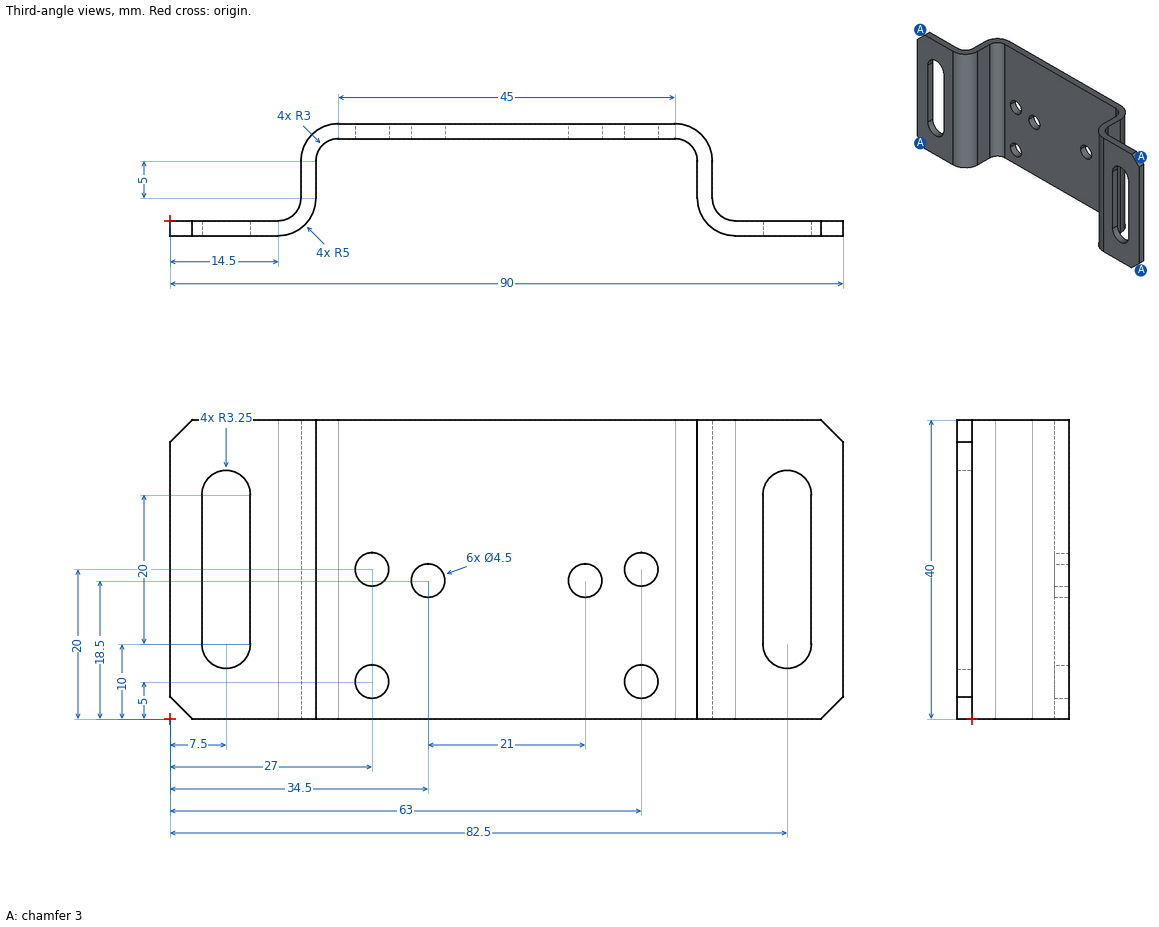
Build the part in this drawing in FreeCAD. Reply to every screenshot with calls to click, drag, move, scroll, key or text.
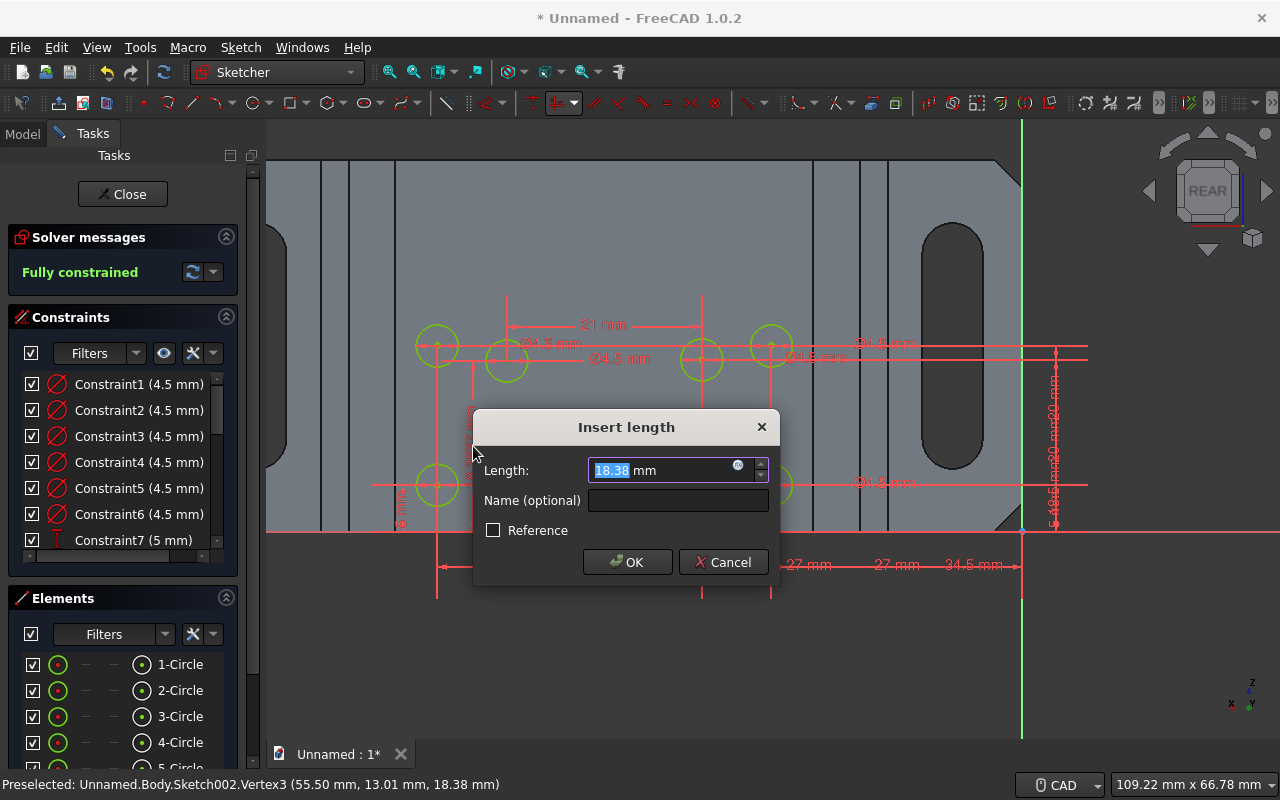
text(18.5)
key(Return)
key(Escape)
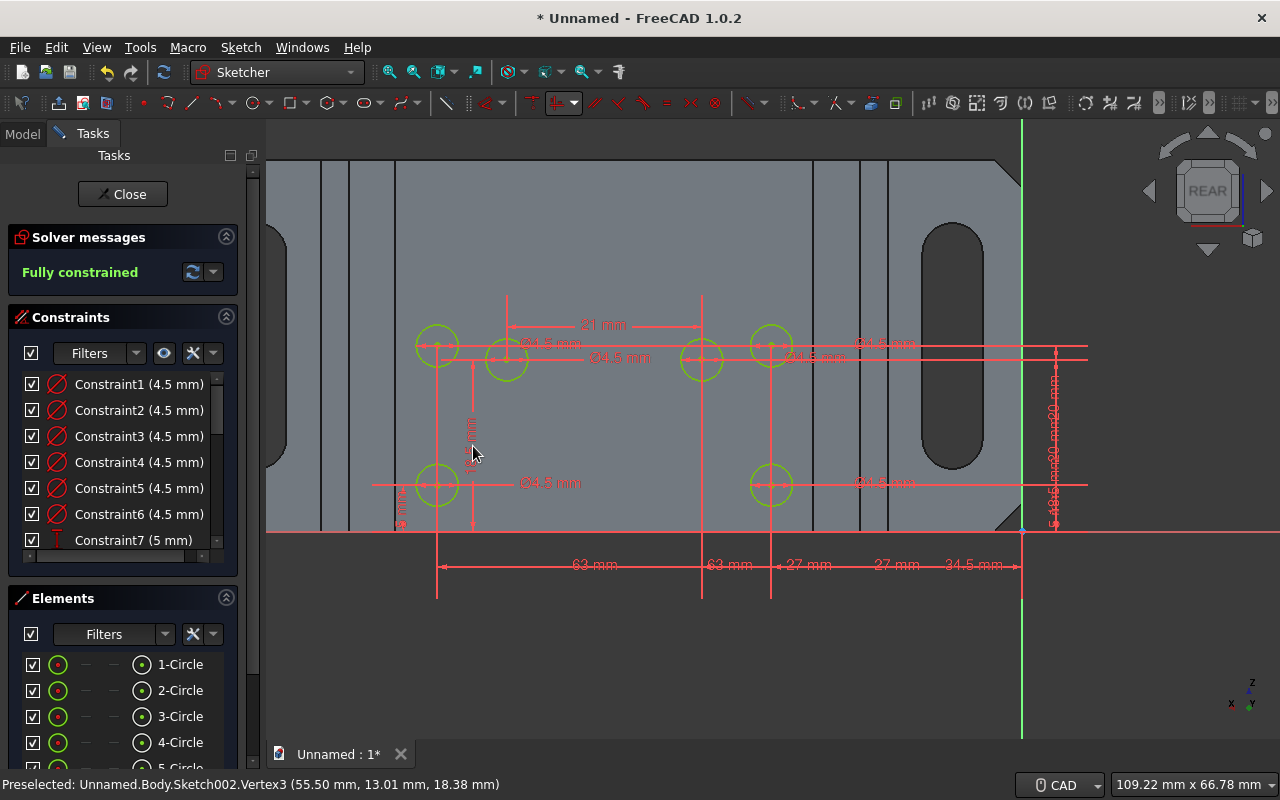
click(123, 194)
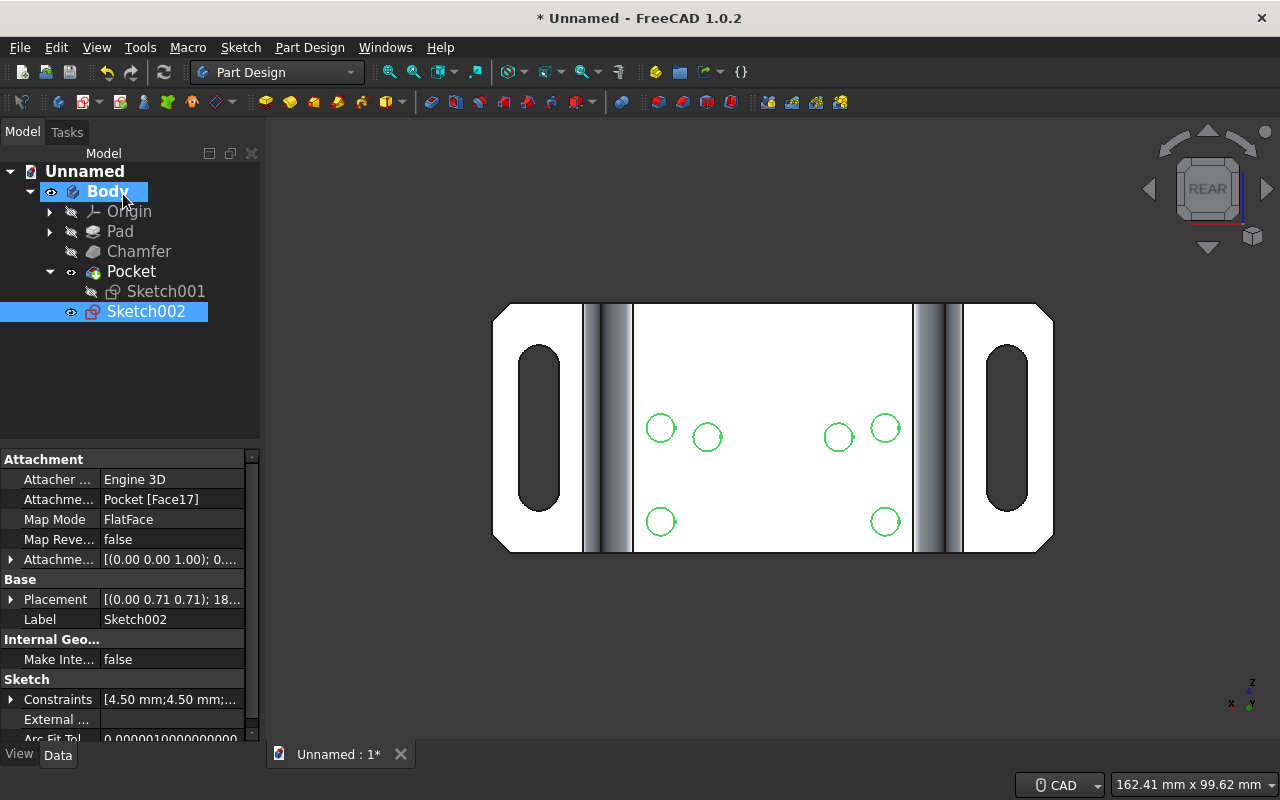
click(432, 102)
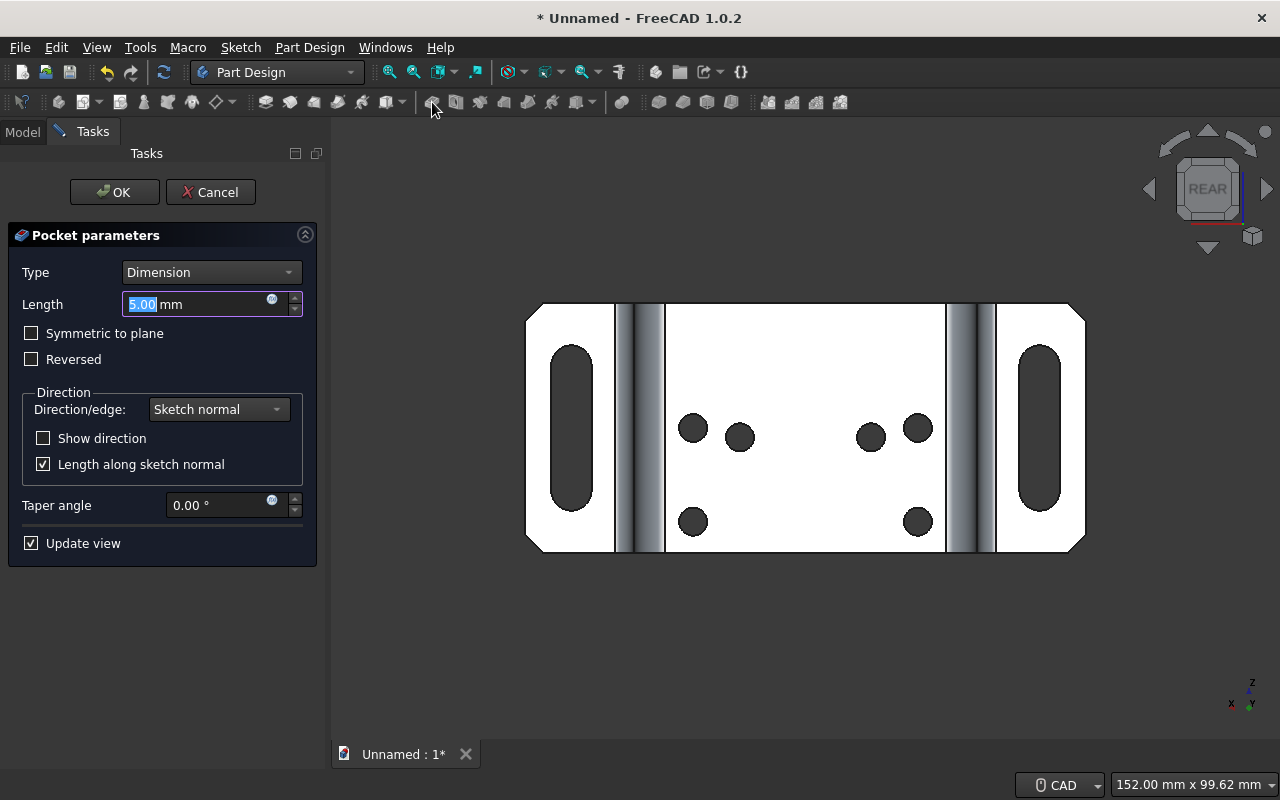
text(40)
key(Tab)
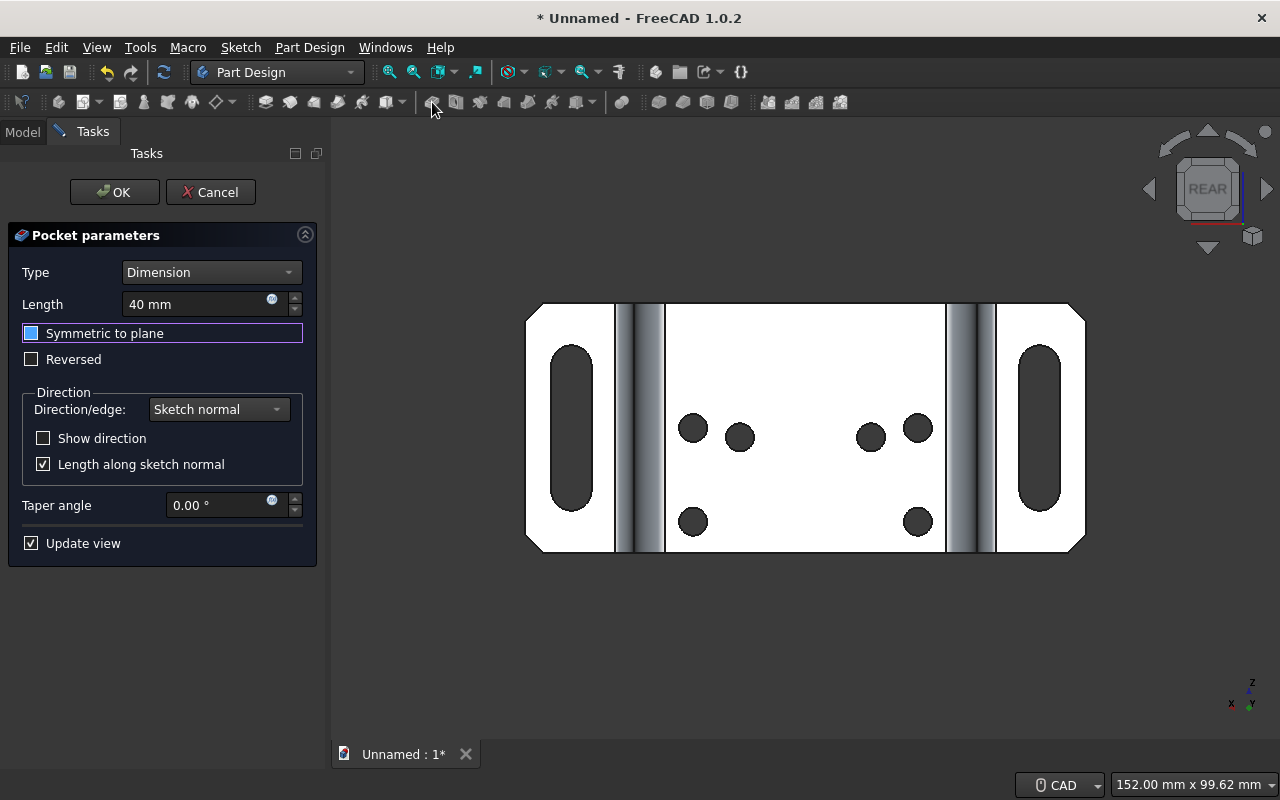
click(115, 192)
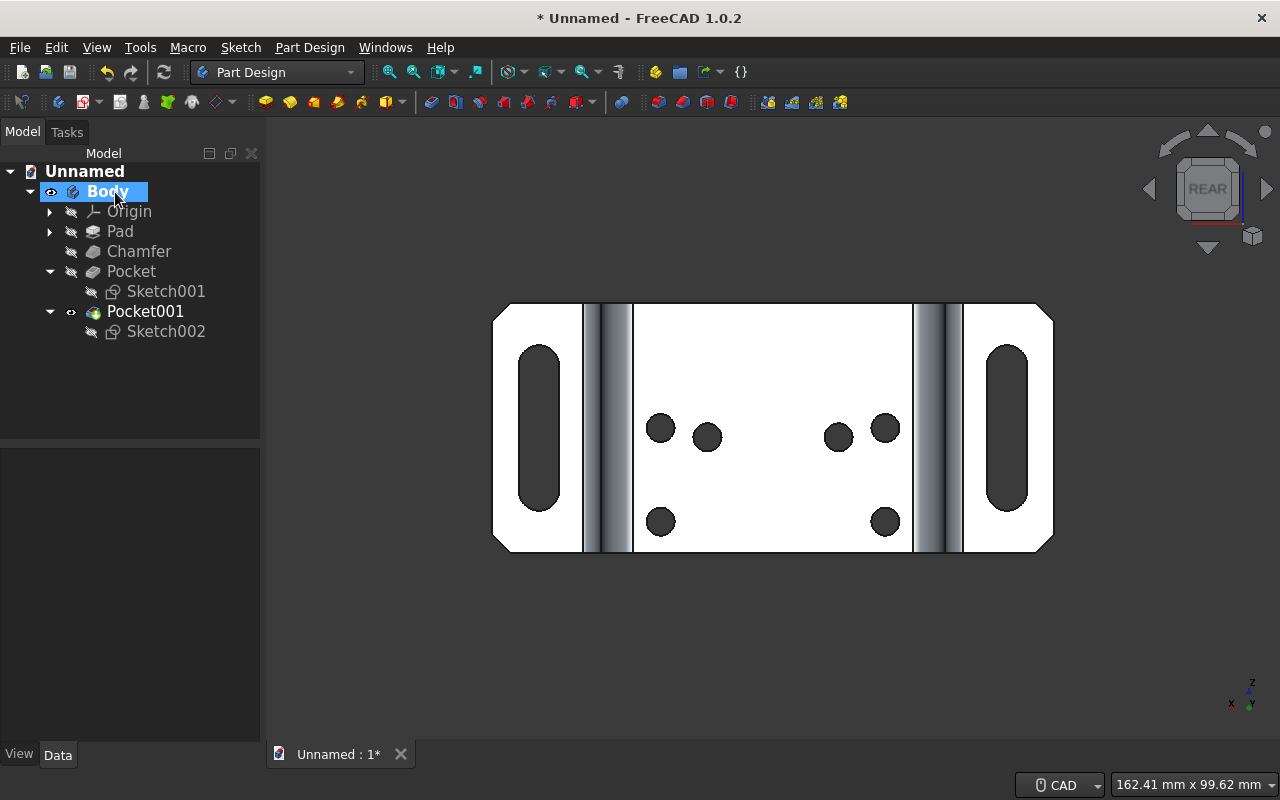
key(0)